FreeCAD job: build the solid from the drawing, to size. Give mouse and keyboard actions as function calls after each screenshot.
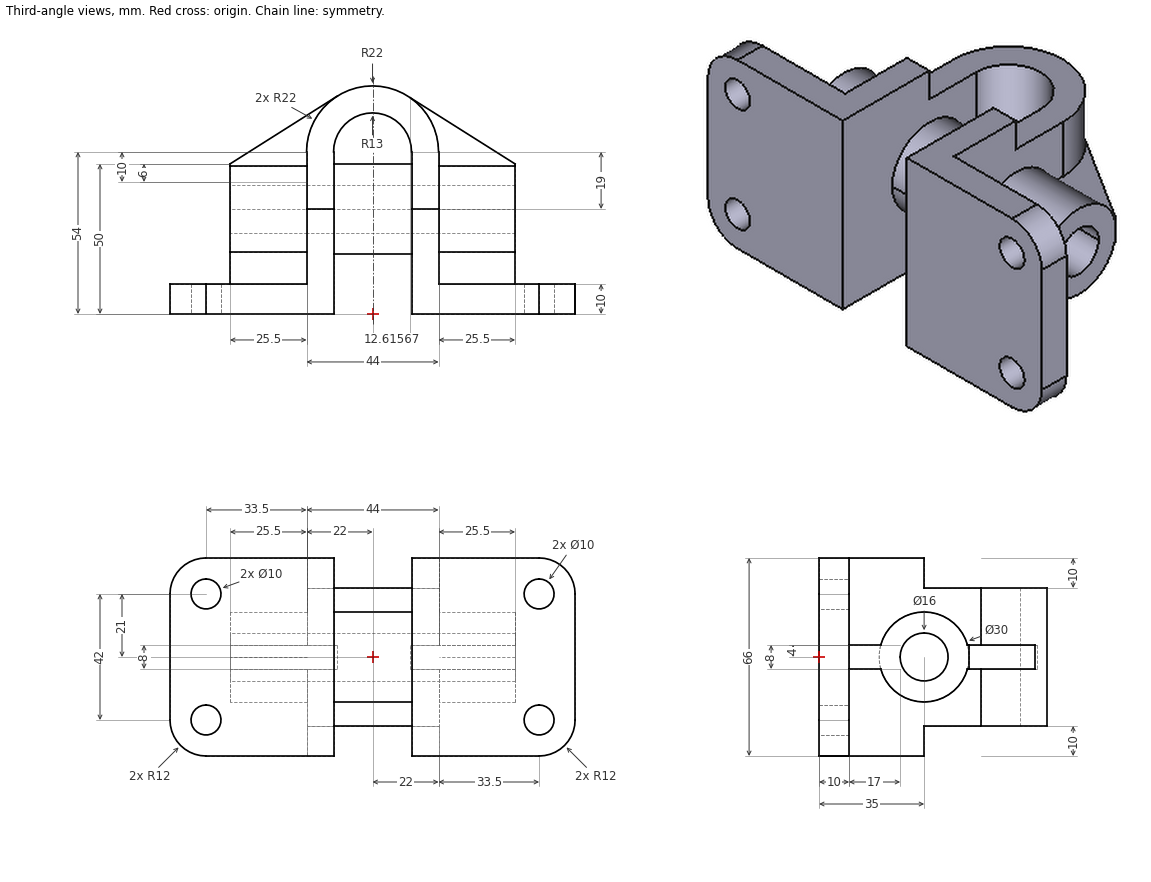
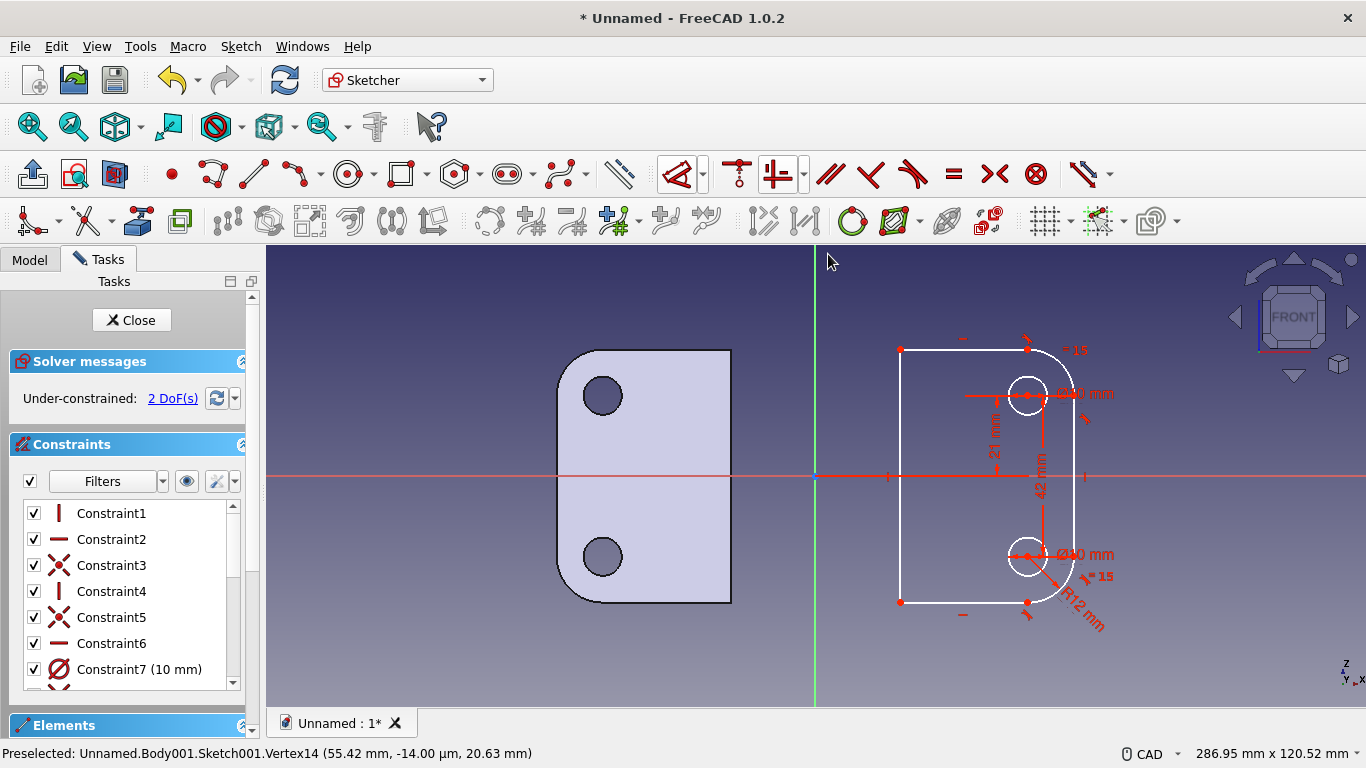
click(900, 603)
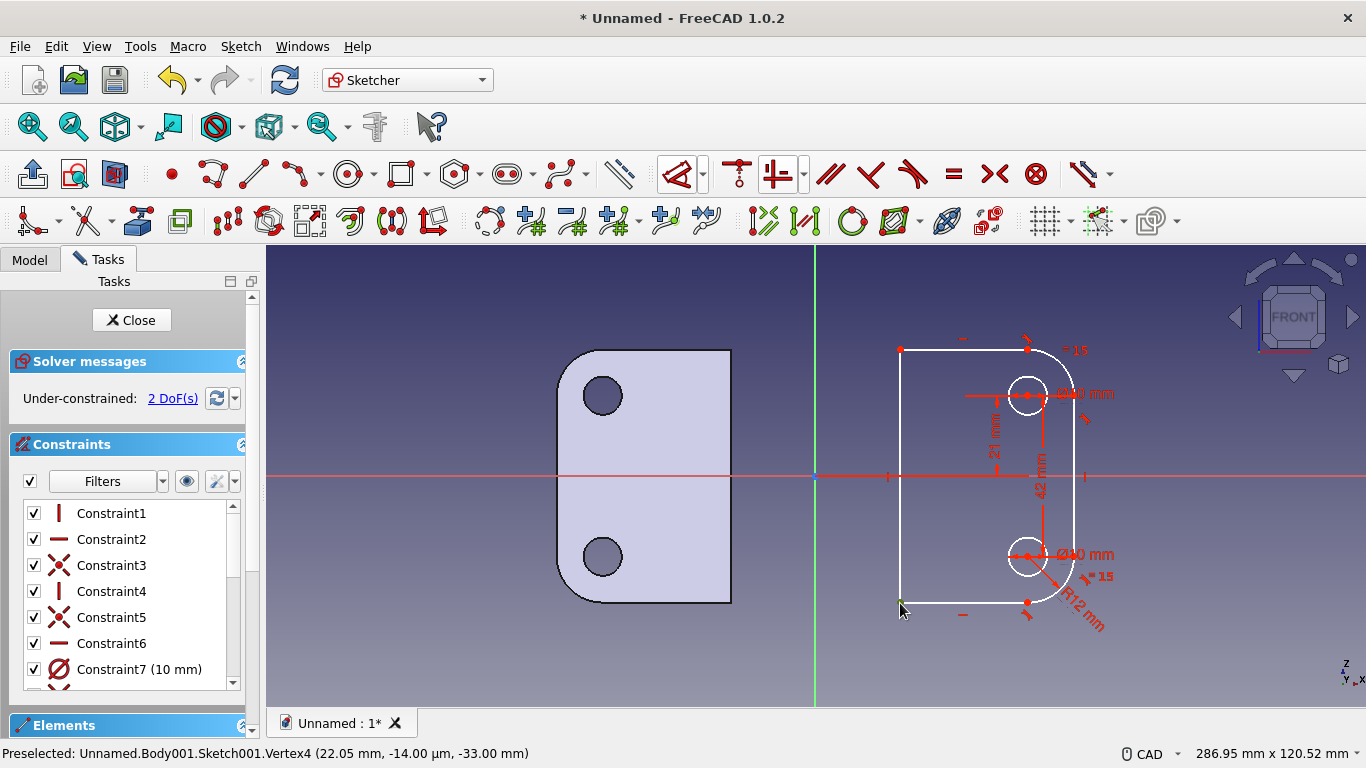
key(l)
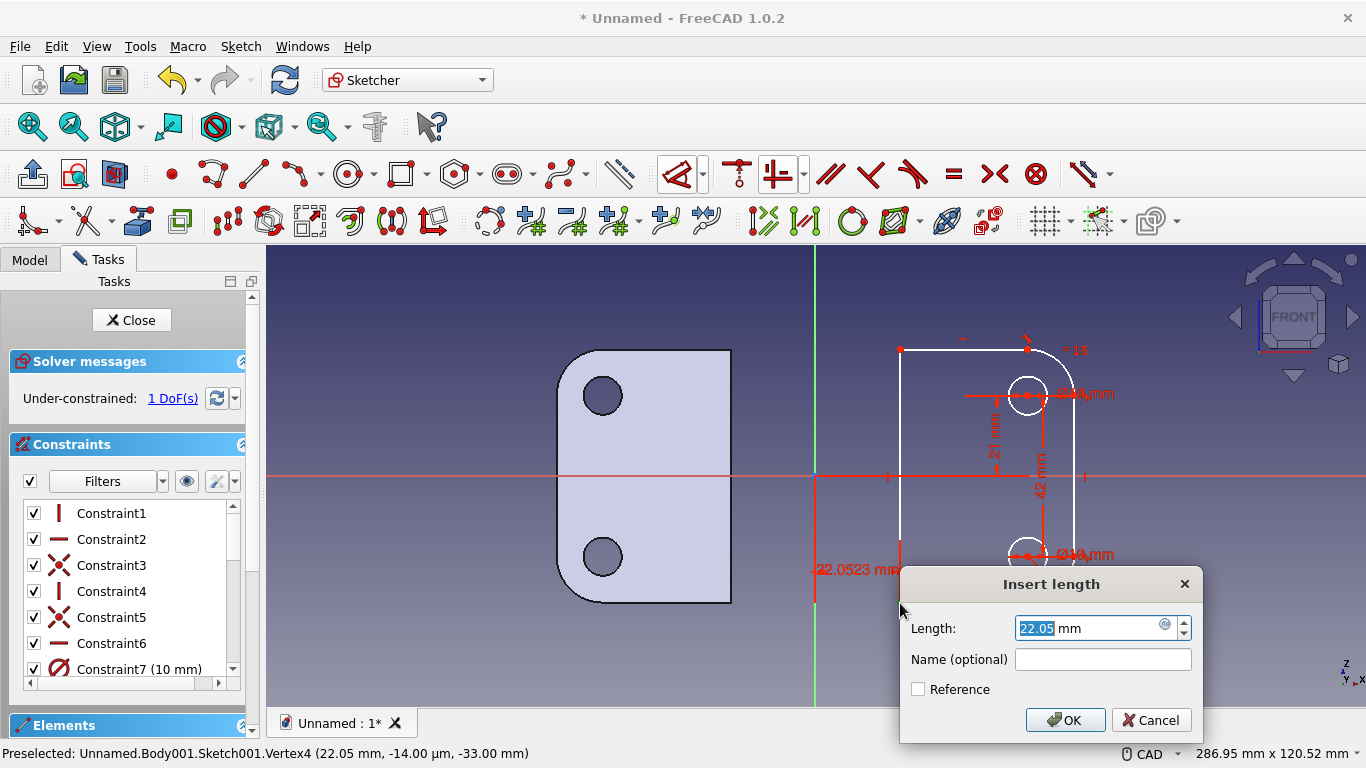
text(22)
key(Return)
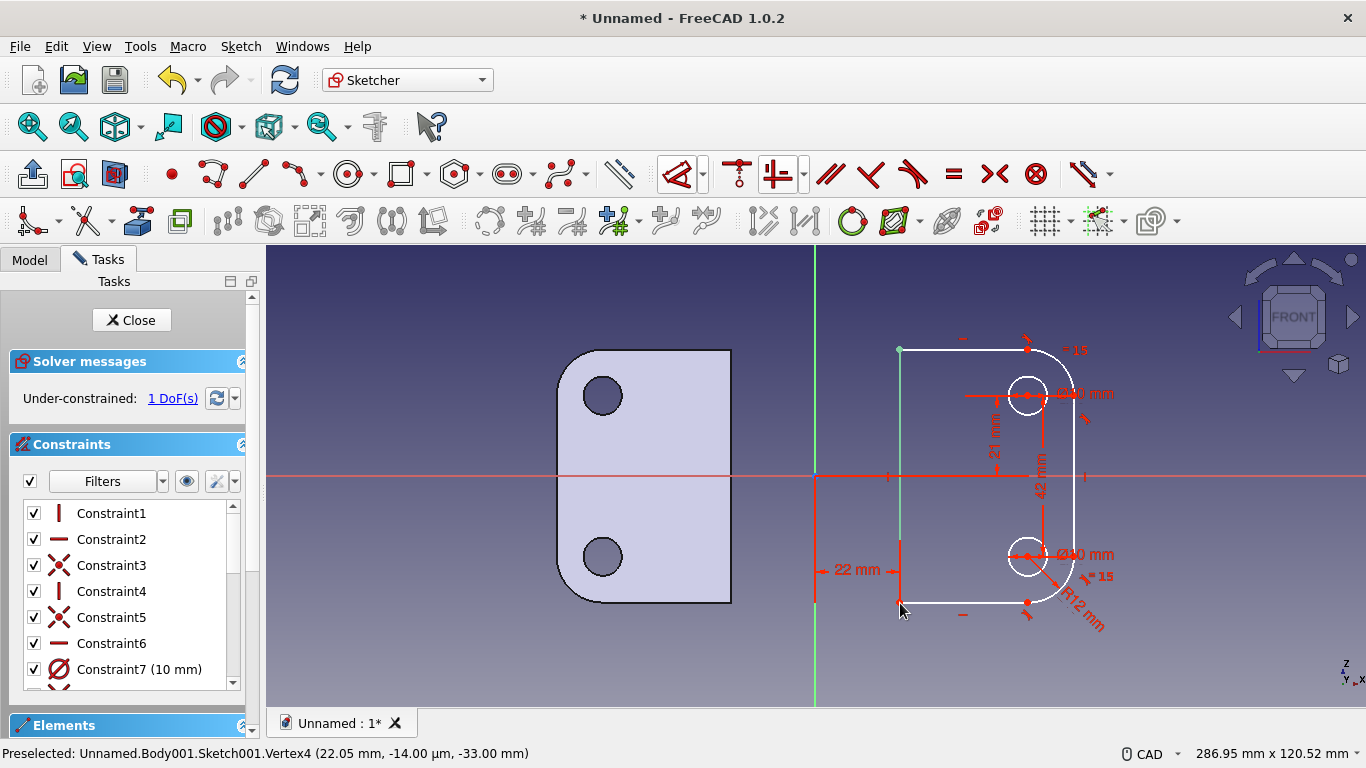
click(989, 603)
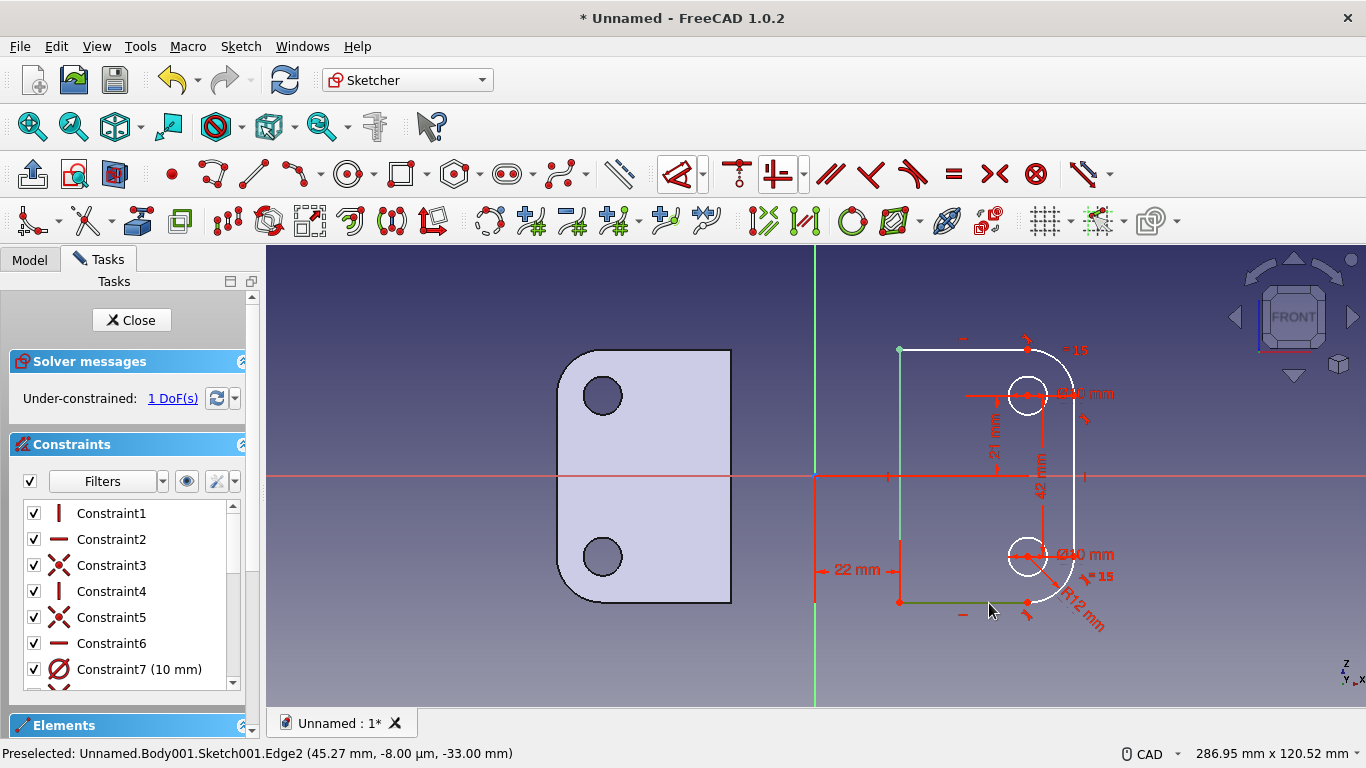
key(l)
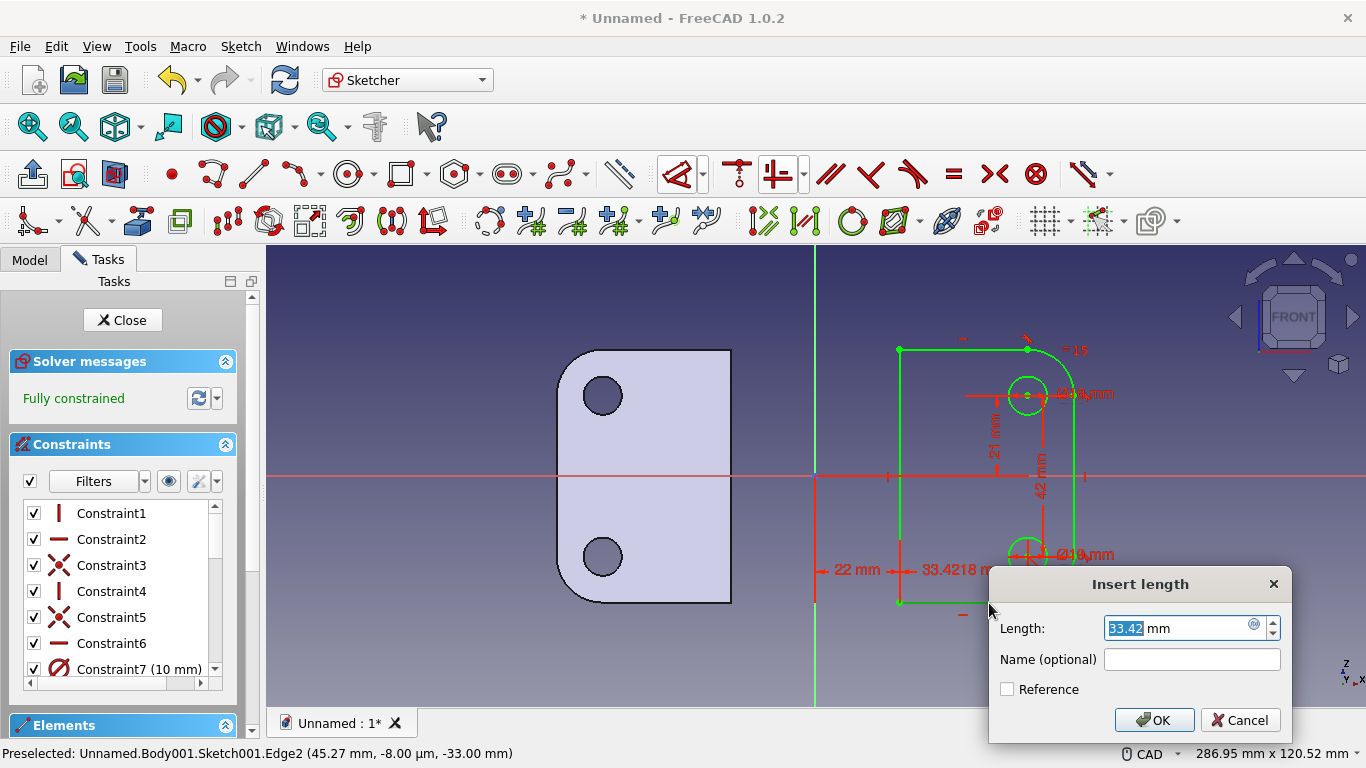
text(33.5)
key(Return)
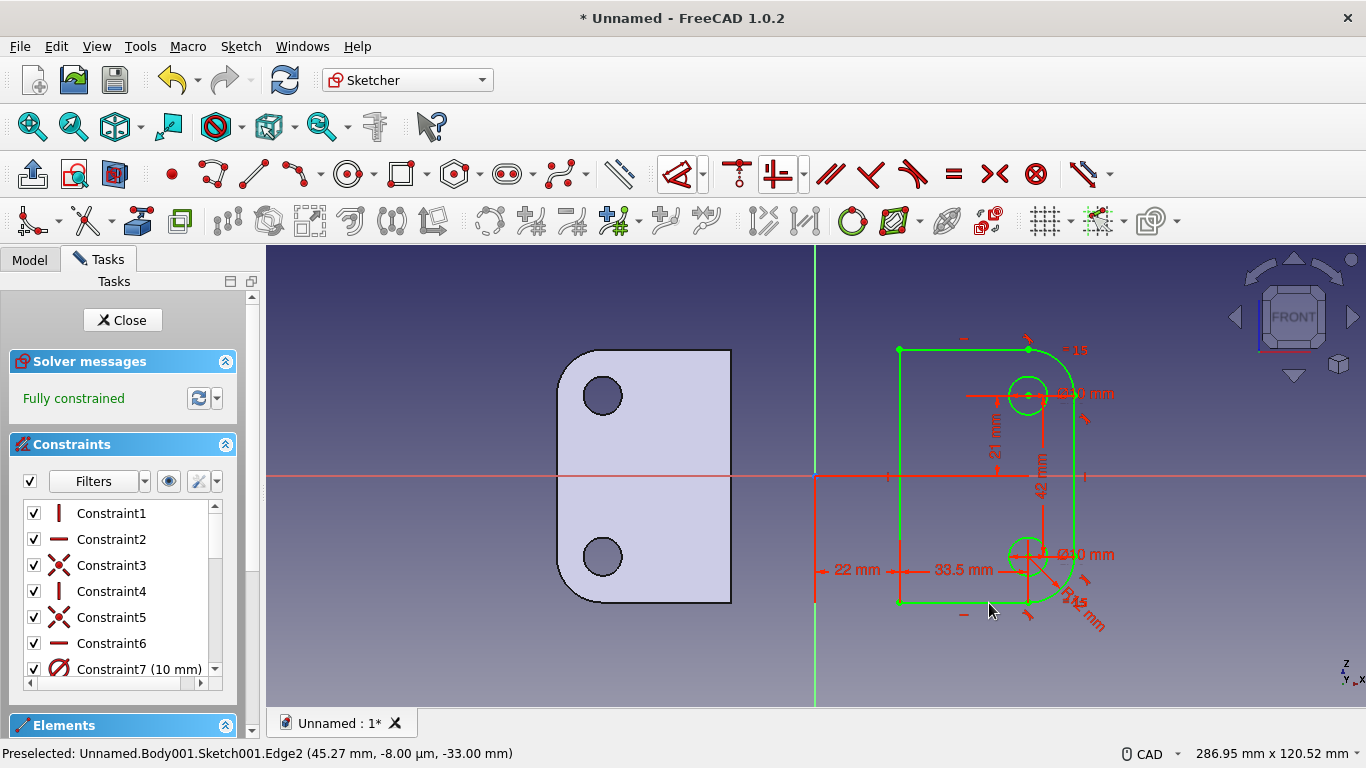
click(123, 320)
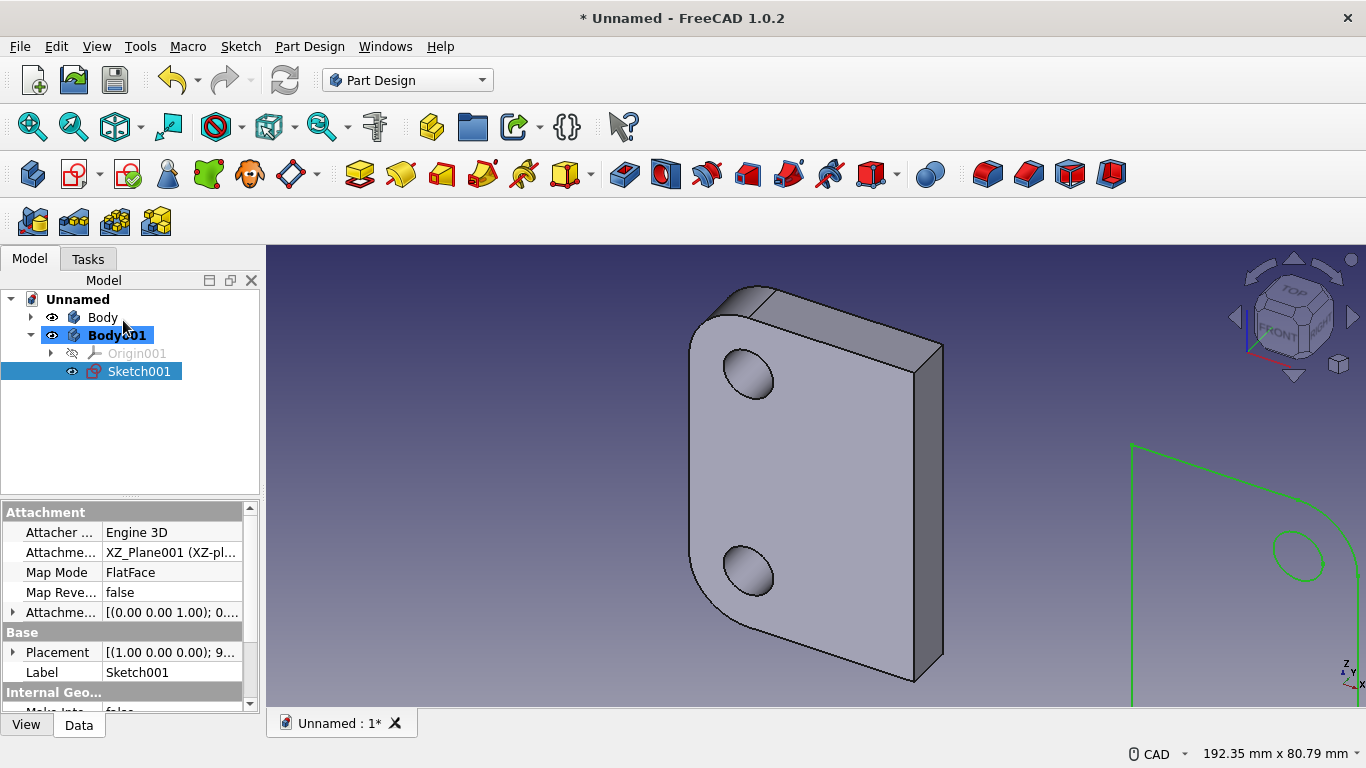
click(360, 174)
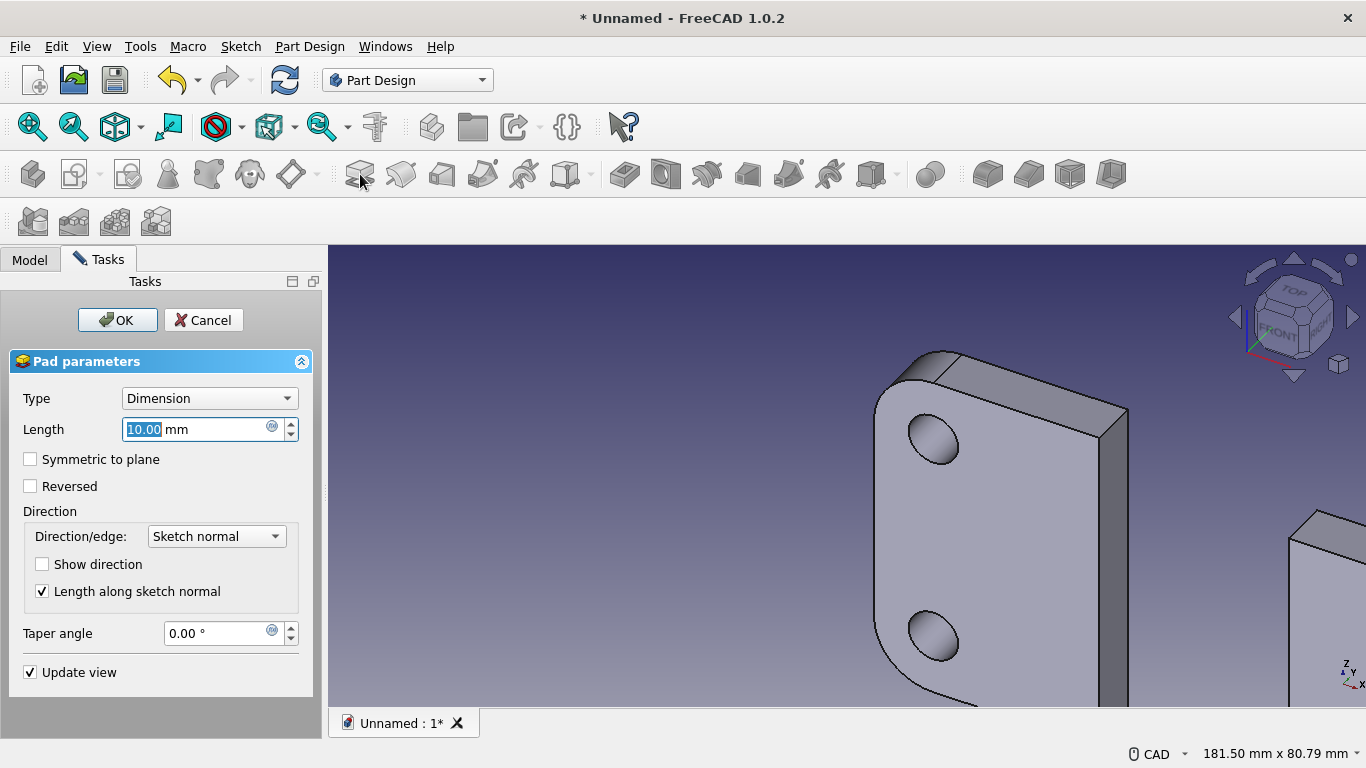
text(10)
key(Tab)